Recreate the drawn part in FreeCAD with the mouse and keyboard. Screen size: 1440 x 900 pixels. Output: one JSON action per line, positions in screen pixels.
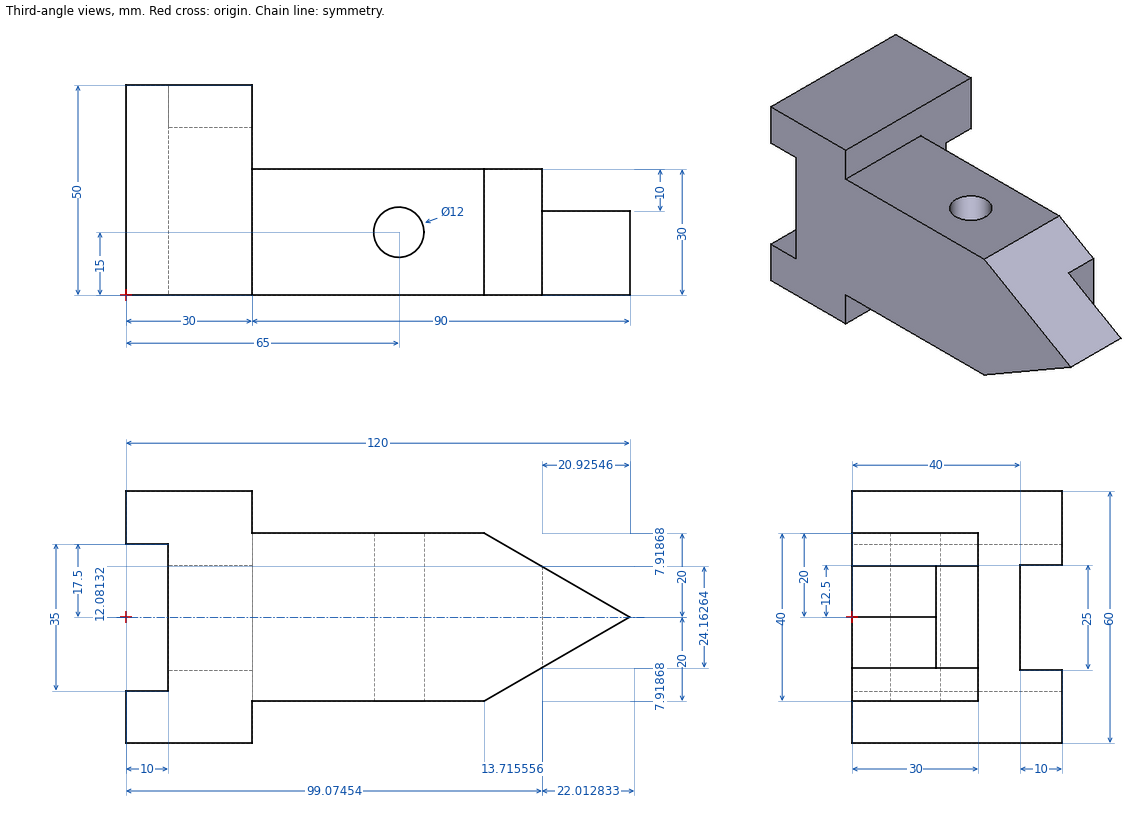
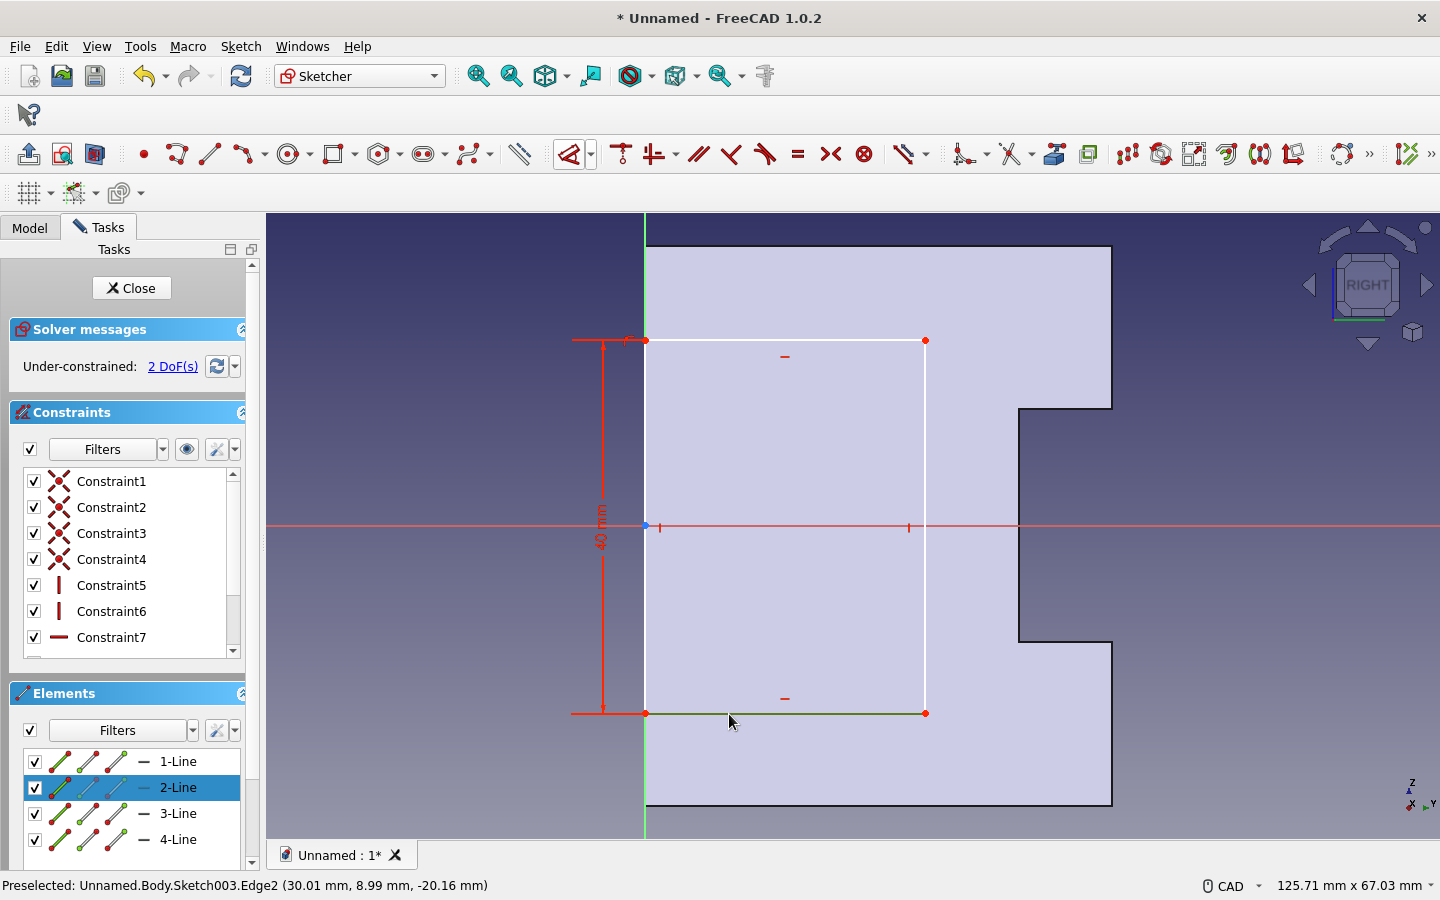
{"action": "left_click", "coordinate": [590, 154]}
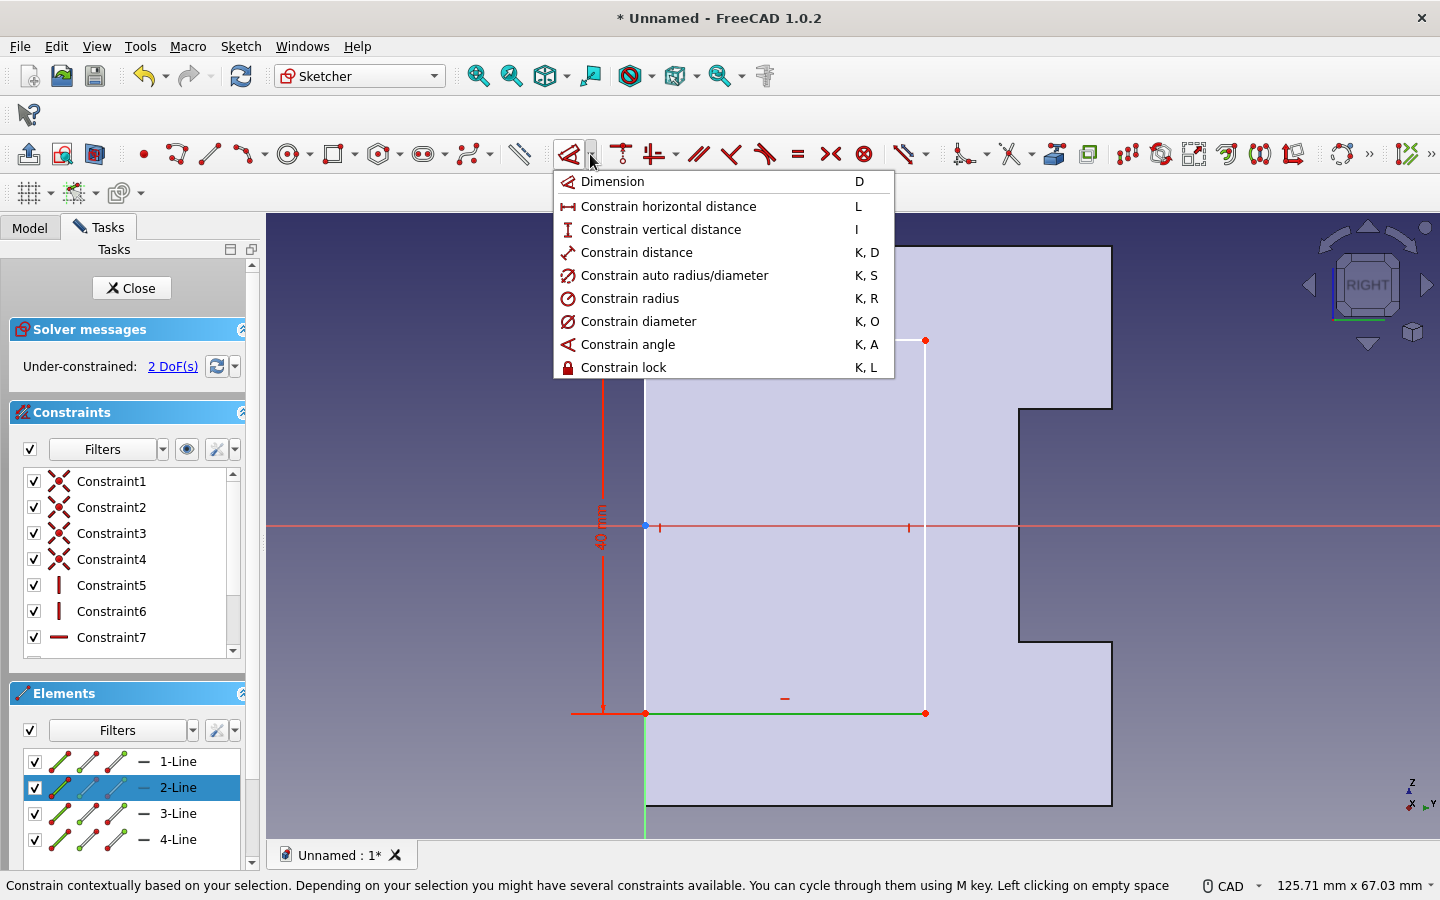
{"action": "left_click", "coordinate": [724, 206]}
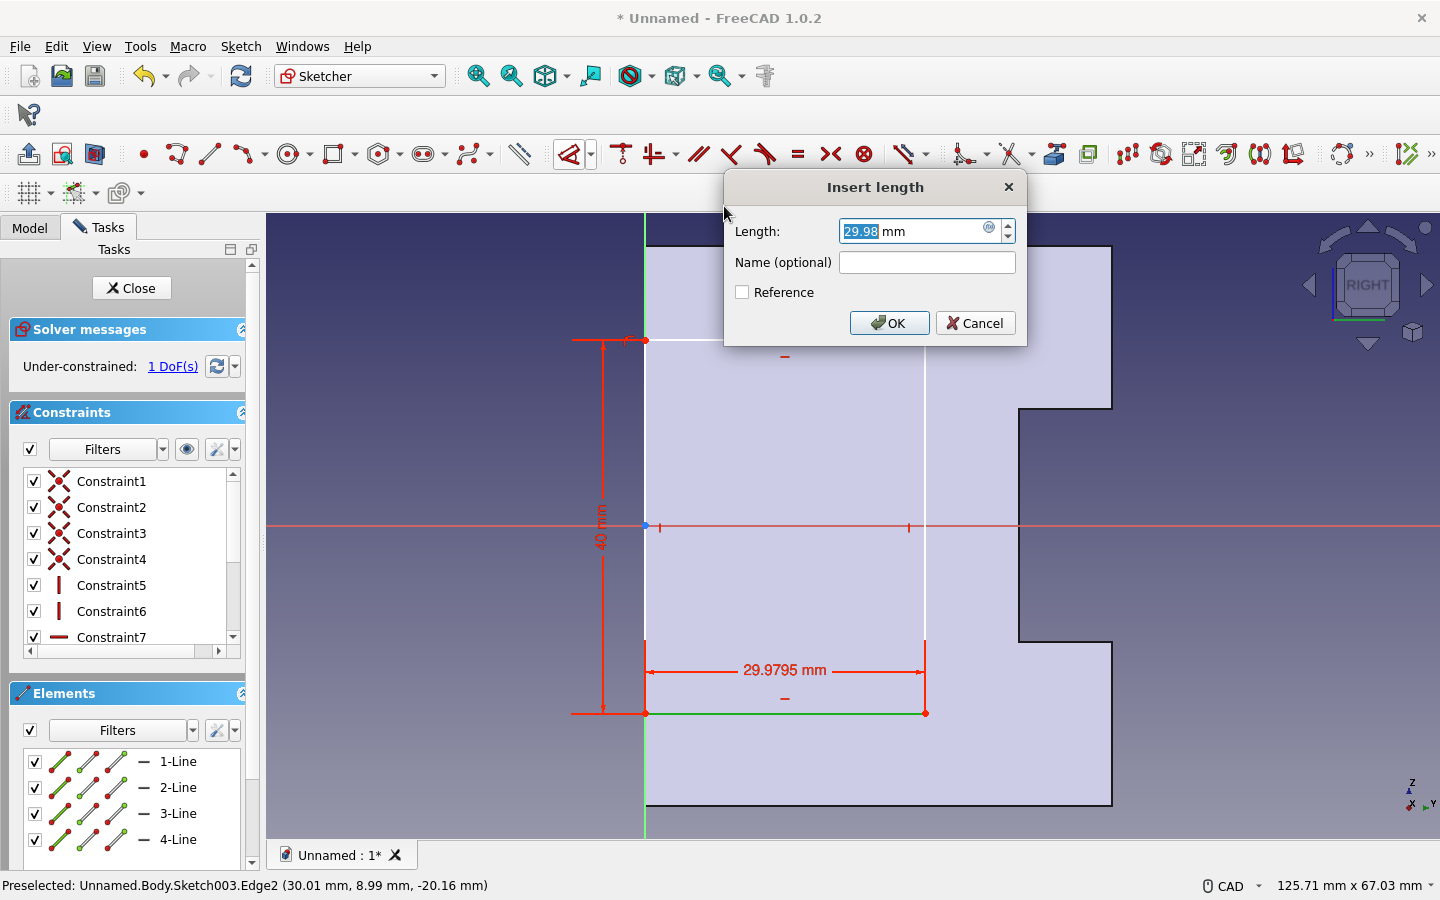
{"action": "type", "text": "30"}
{"action": "key", "text": "Return"}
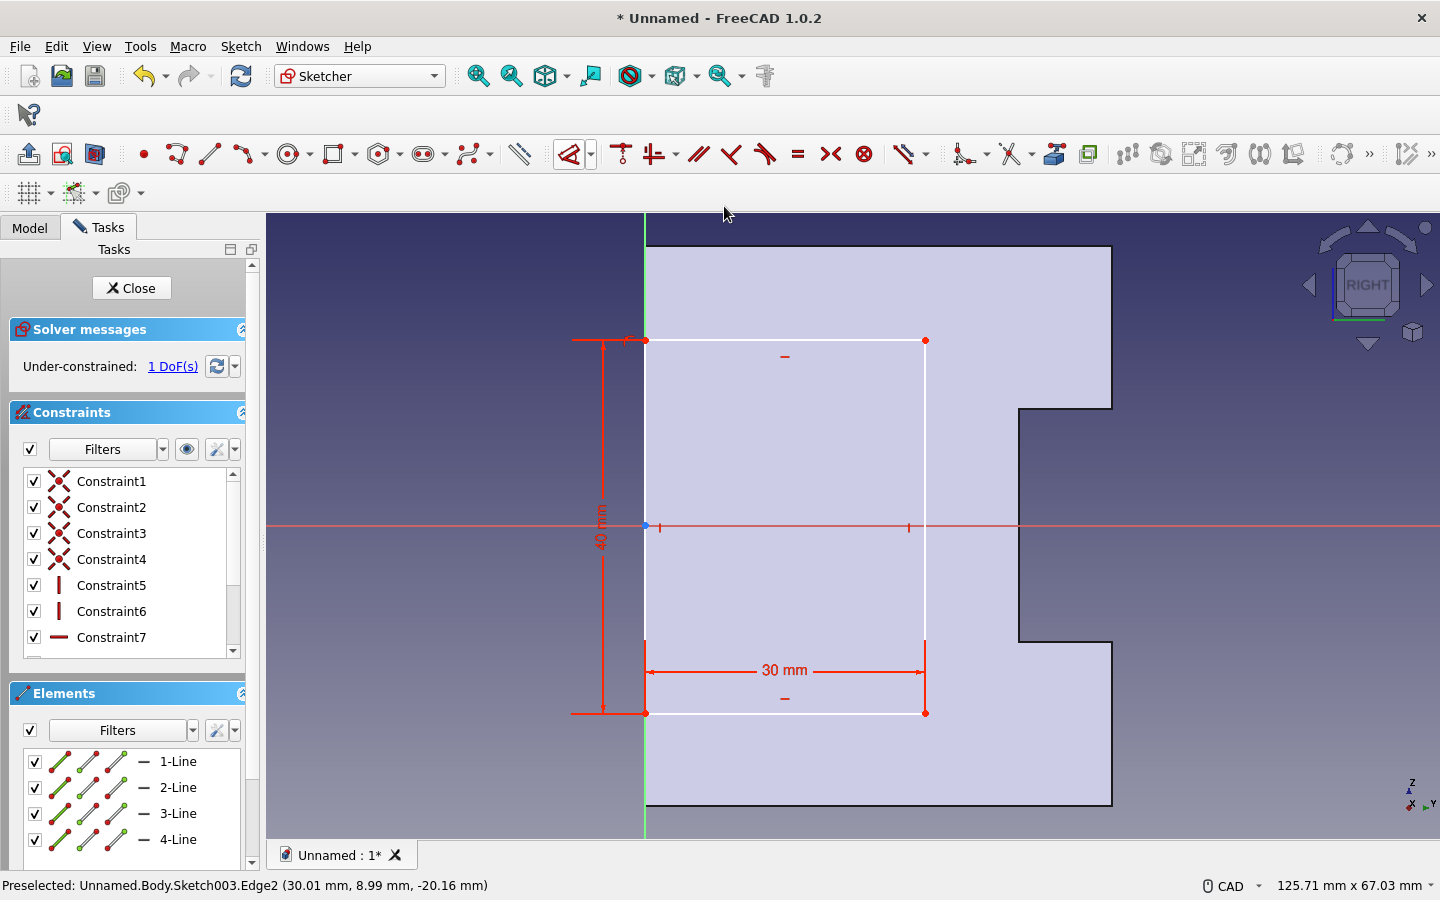
{"action": "left_click", "coordinate": [645, 340]}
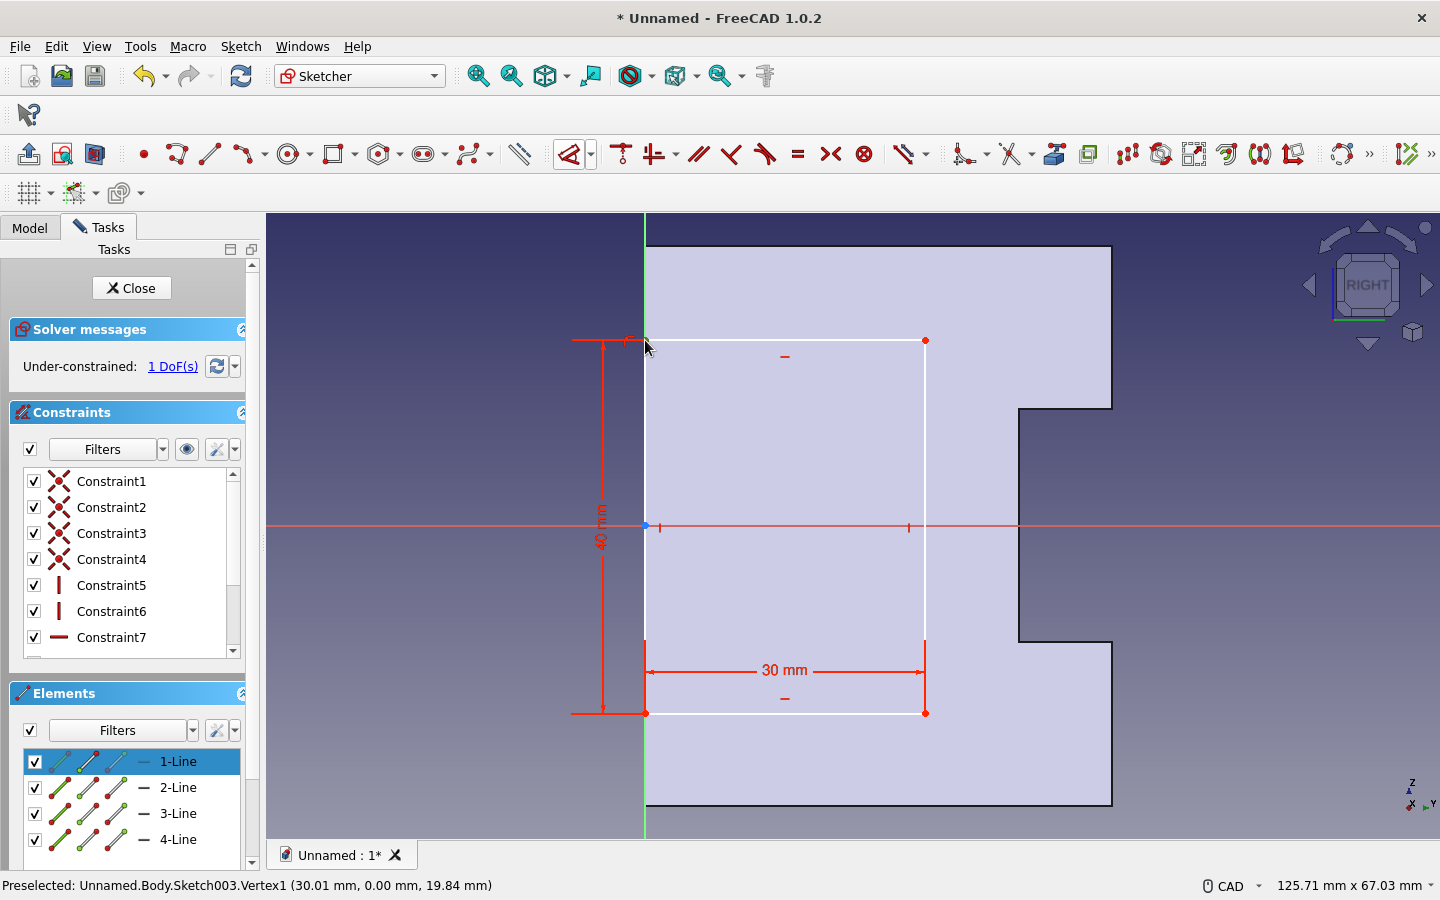
{"action": "key", "text": "i"}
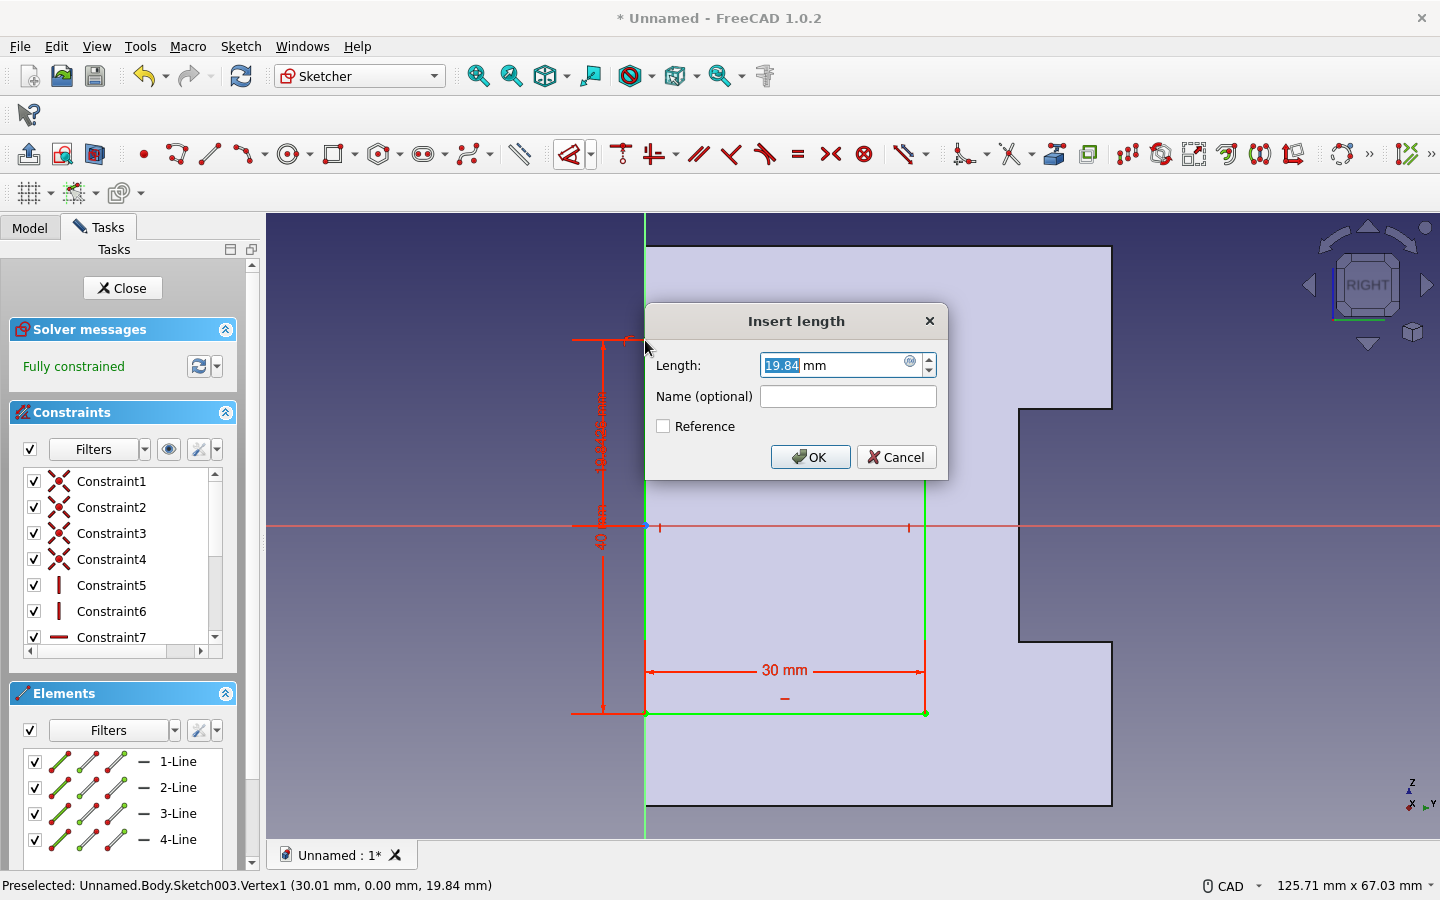
{"action": "type", "text": "20"}
{"action": "key", "text": "Return"}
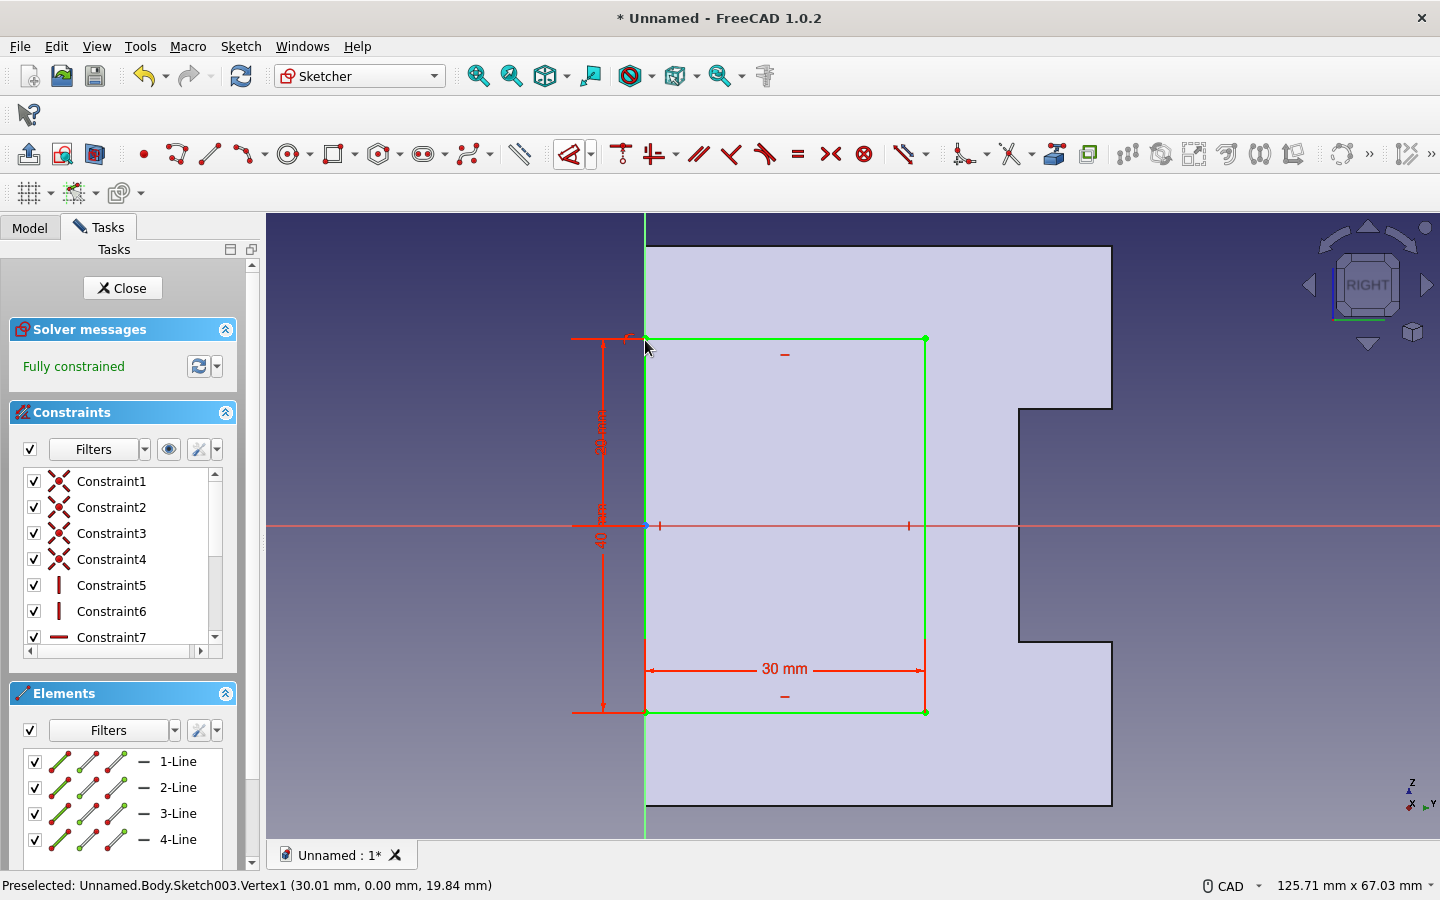
{"action": "left_click", "coordinate": [123, 288]}